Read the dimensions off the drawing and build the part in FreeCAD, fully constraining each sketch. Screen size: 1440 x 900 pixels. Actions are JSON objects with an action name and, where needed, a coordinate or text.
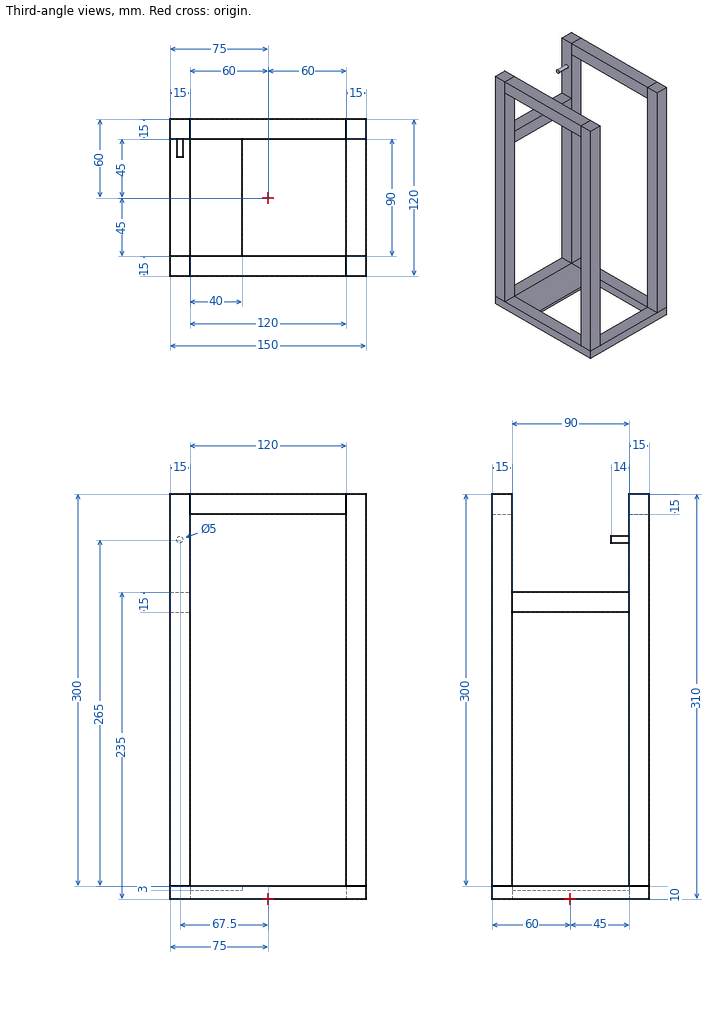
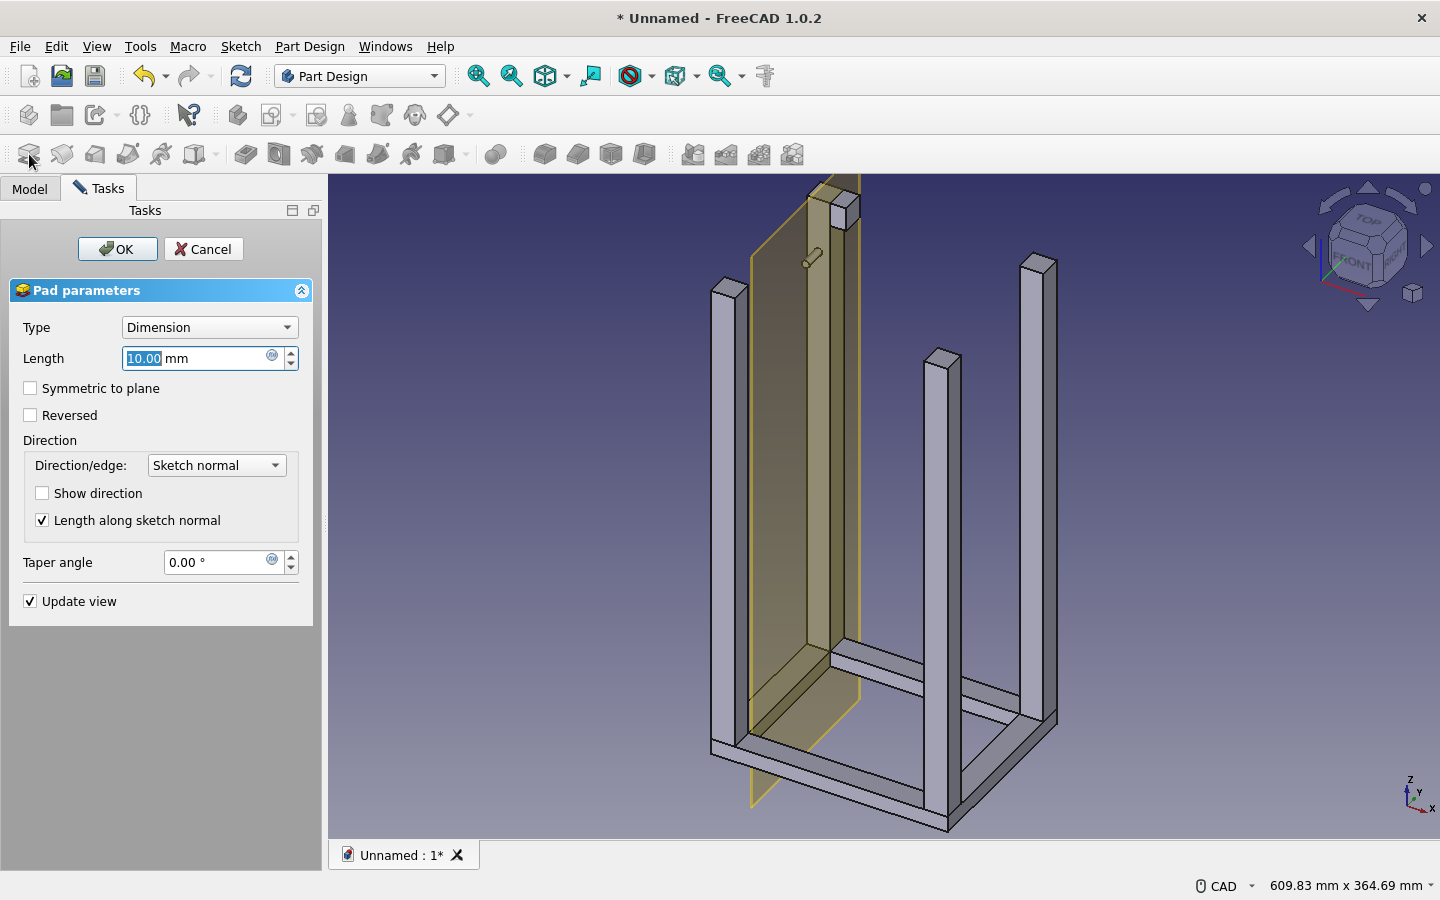
{"action": "type", "text": "120"}
{"action": "key", "text": "Tab"}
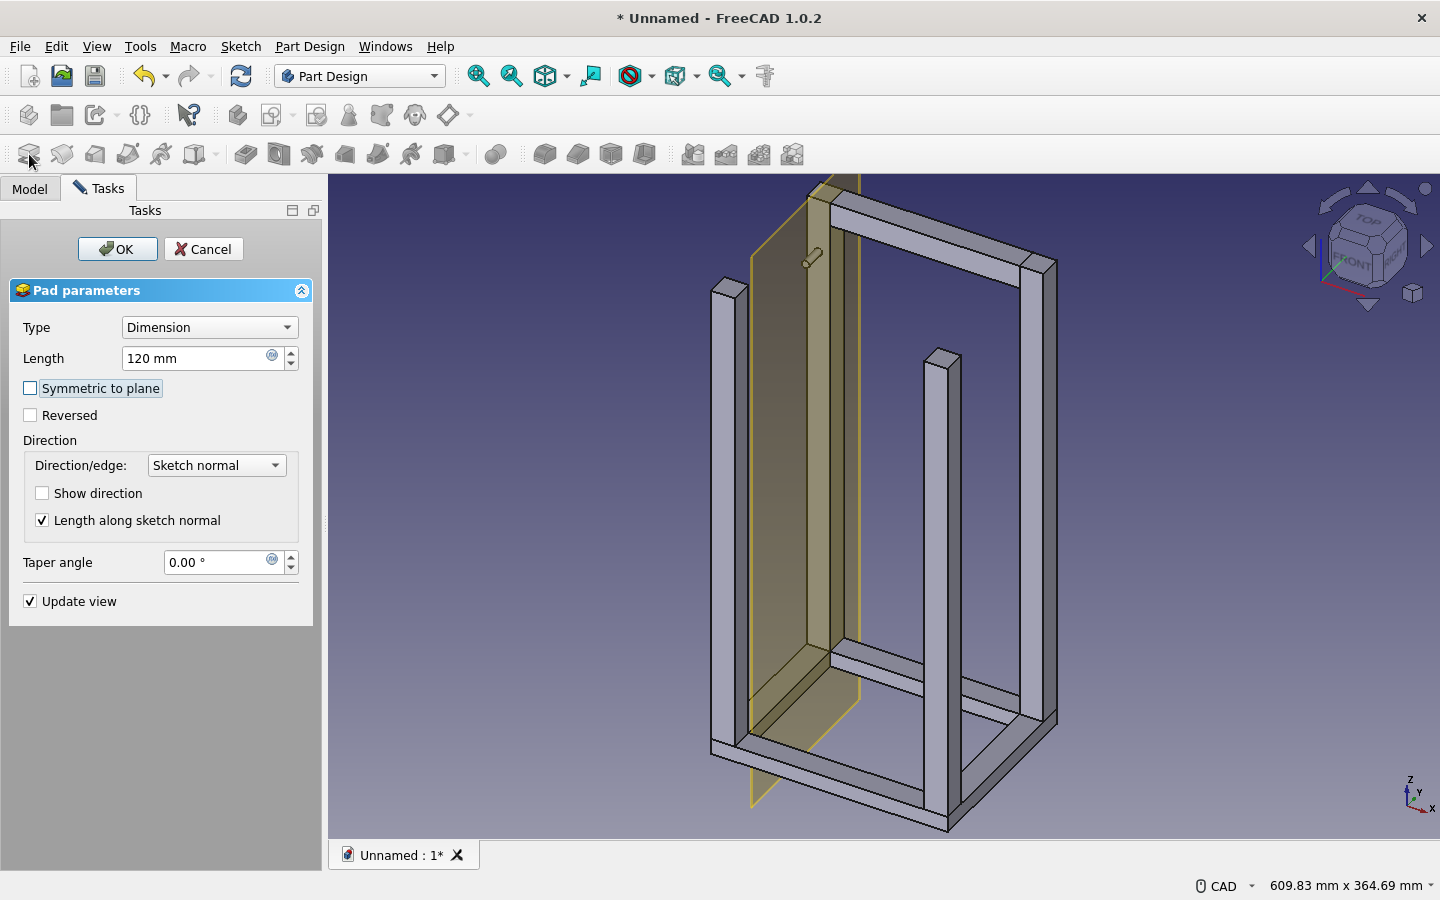
{"action": "left_click", "coordinate": [118, 249]}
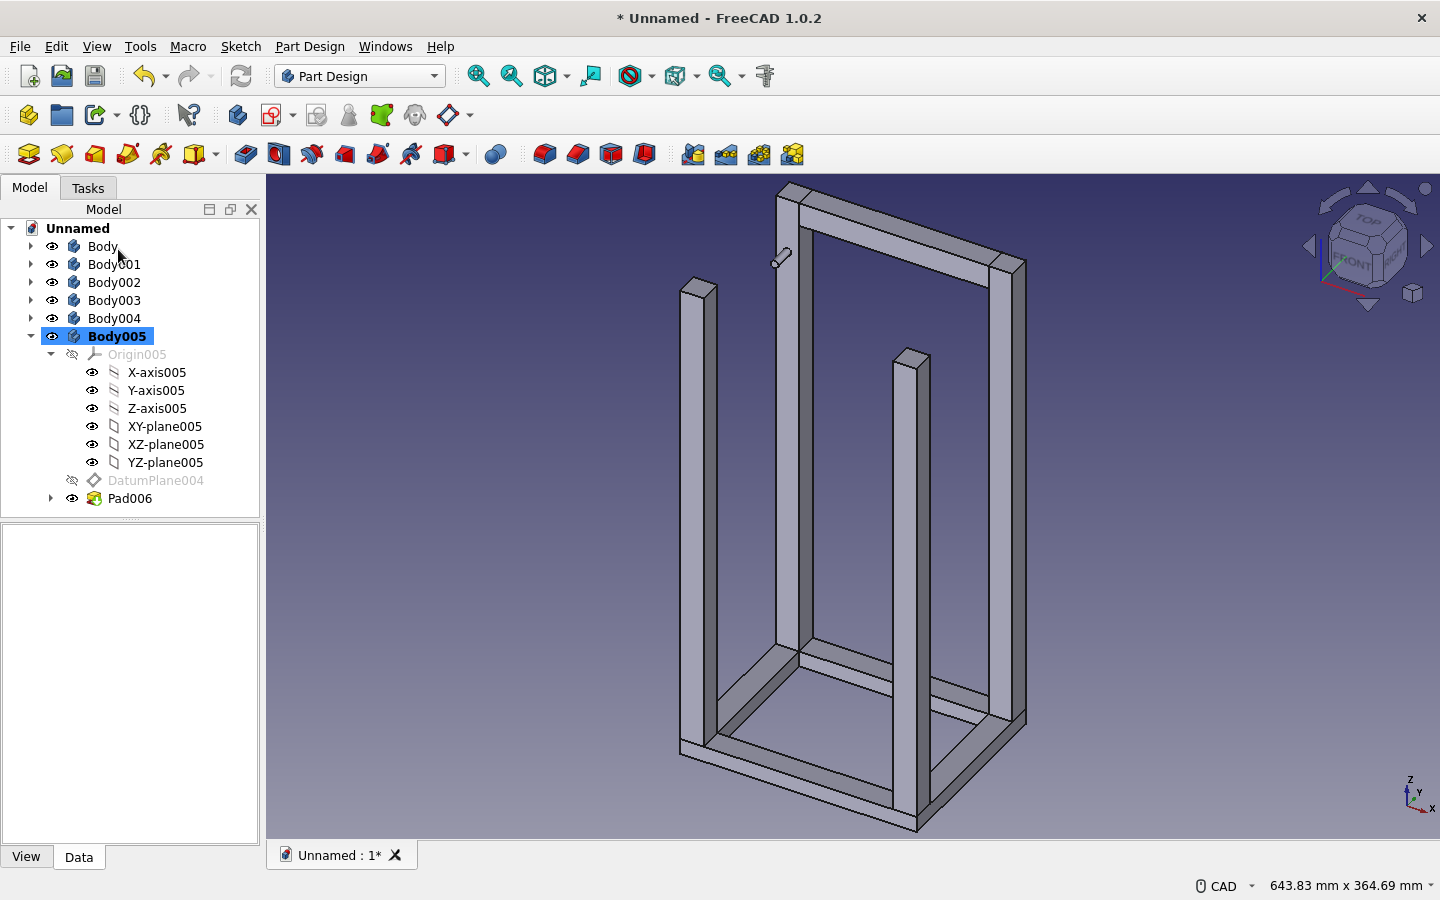
{"action": "left_click", "coordinate": [479, 76]}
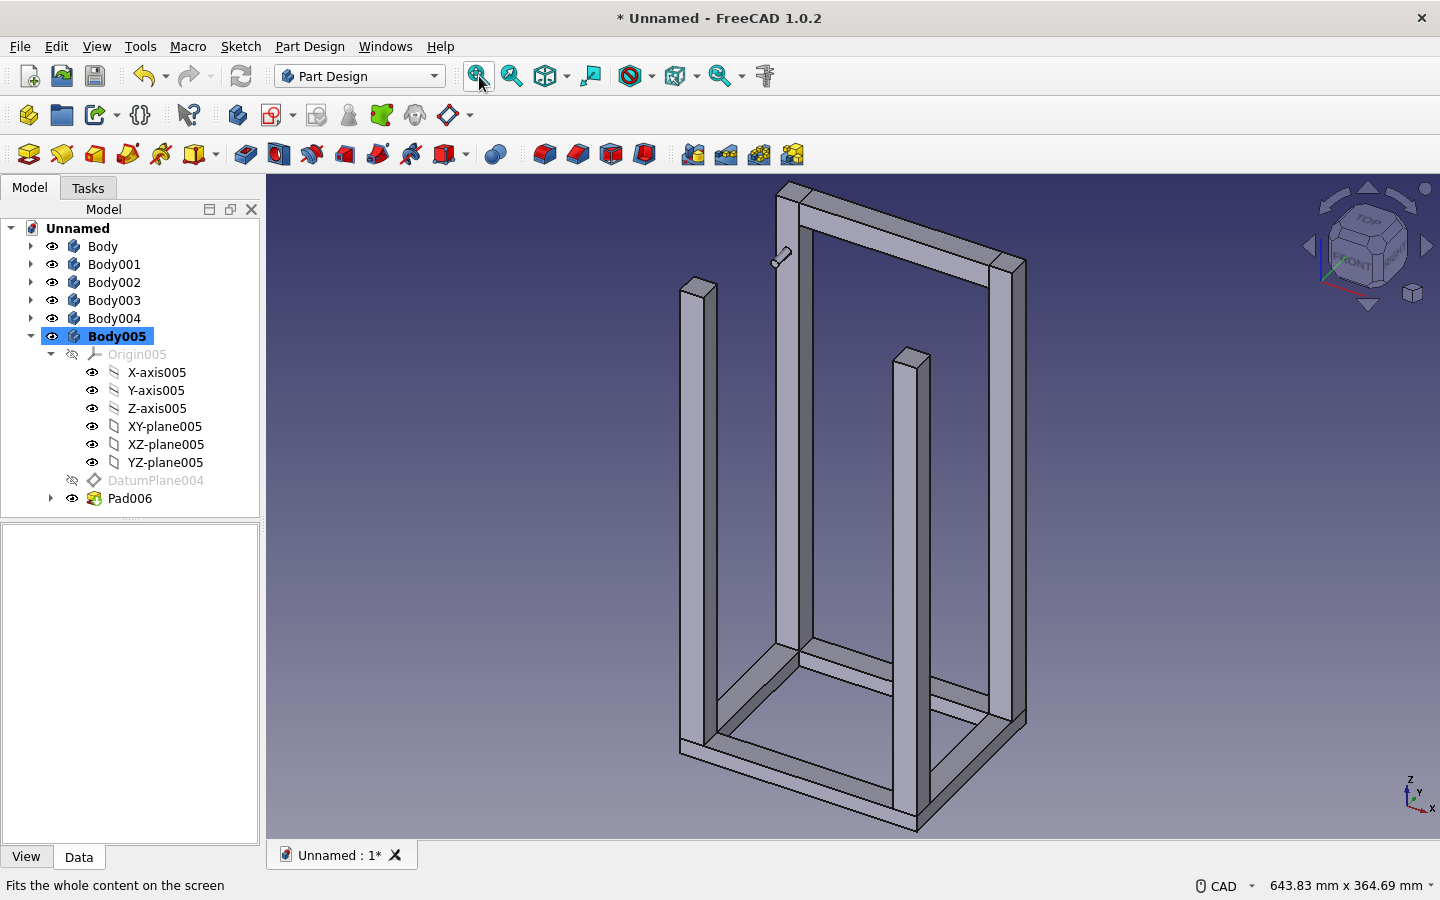
{"action": "left_click", "coordinate": [238, 116]}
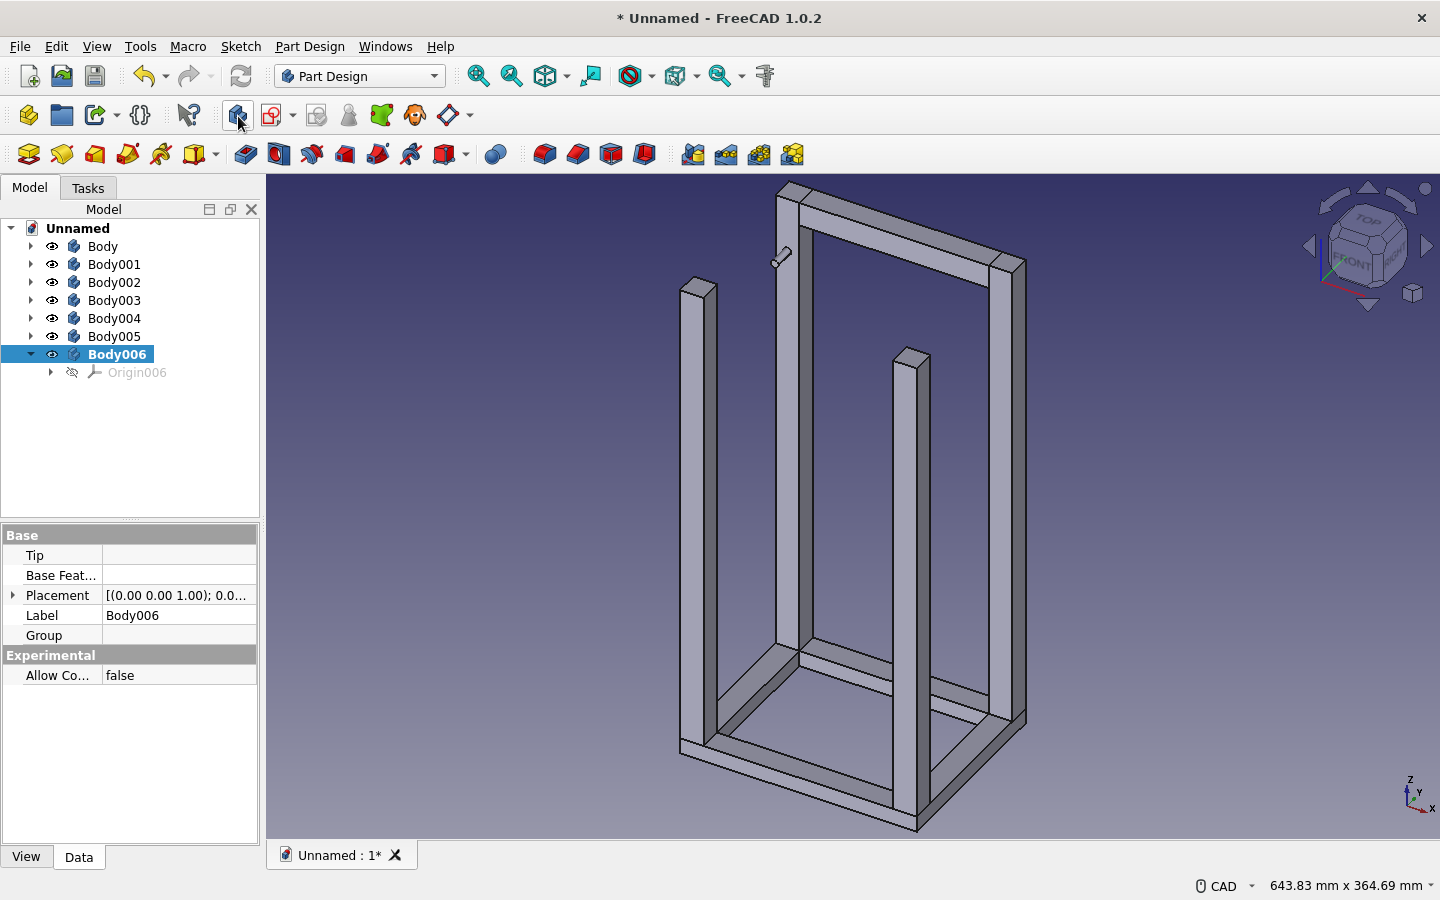
{"action": "left_click", "coordinate": [51, 372]}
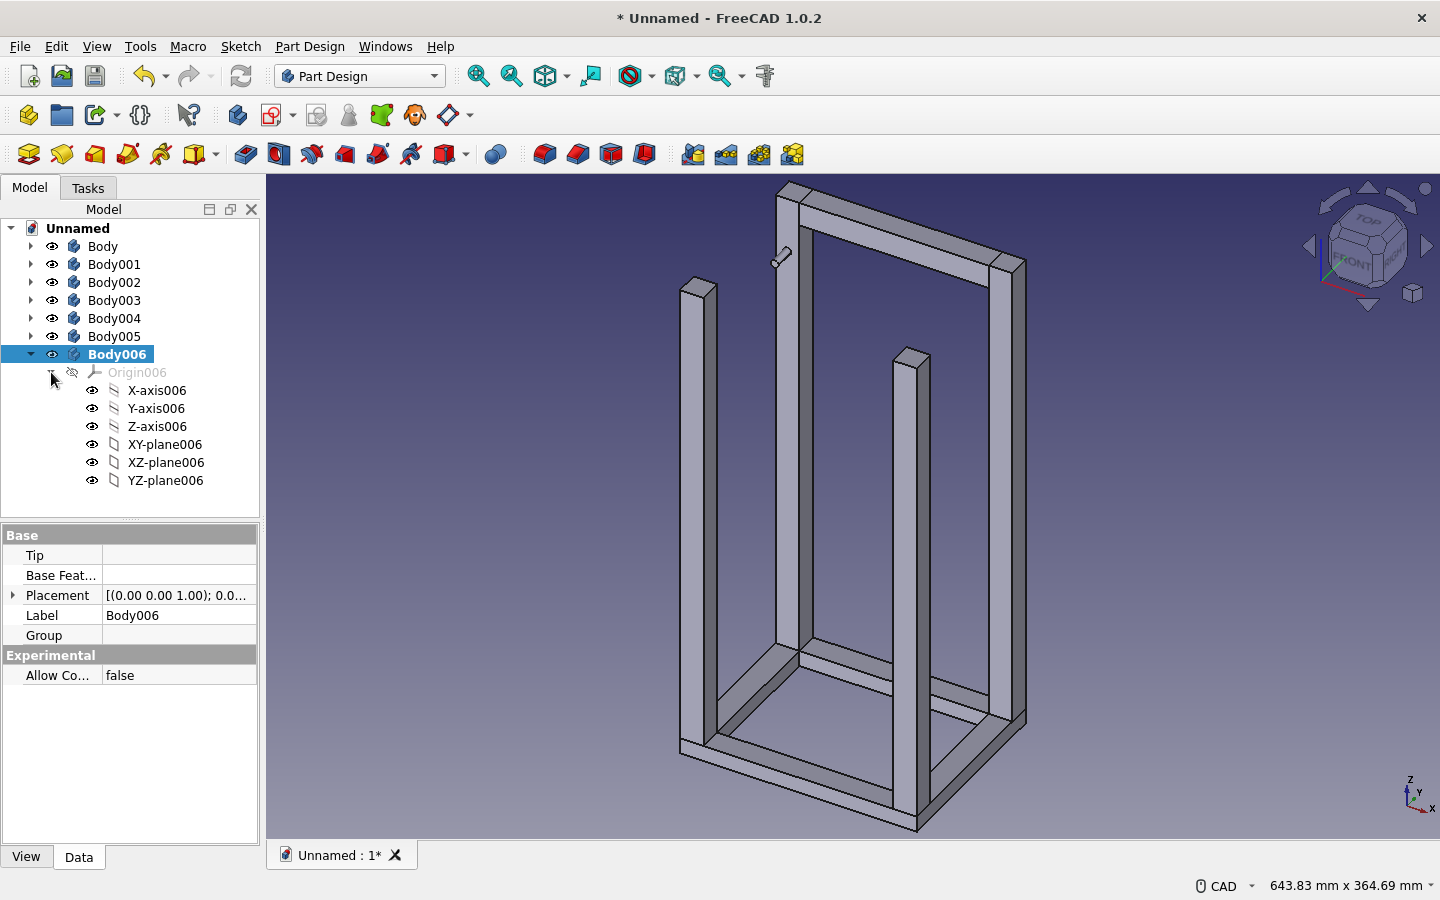
{"action": "left_click", "coordinate": [137, 480]}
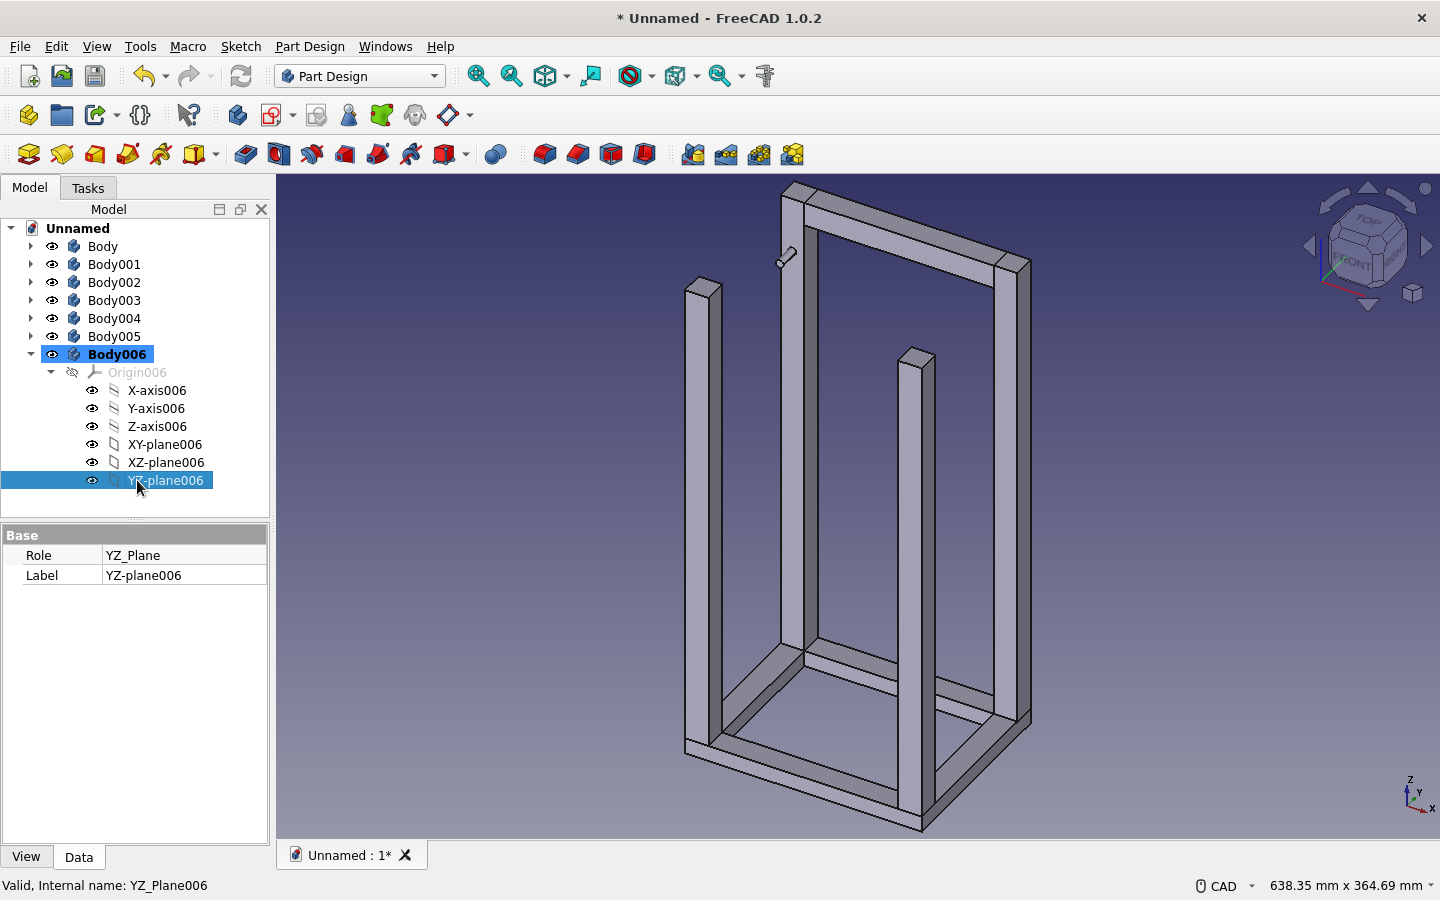
{"action": "left_click", "coordinate": [448, 116]}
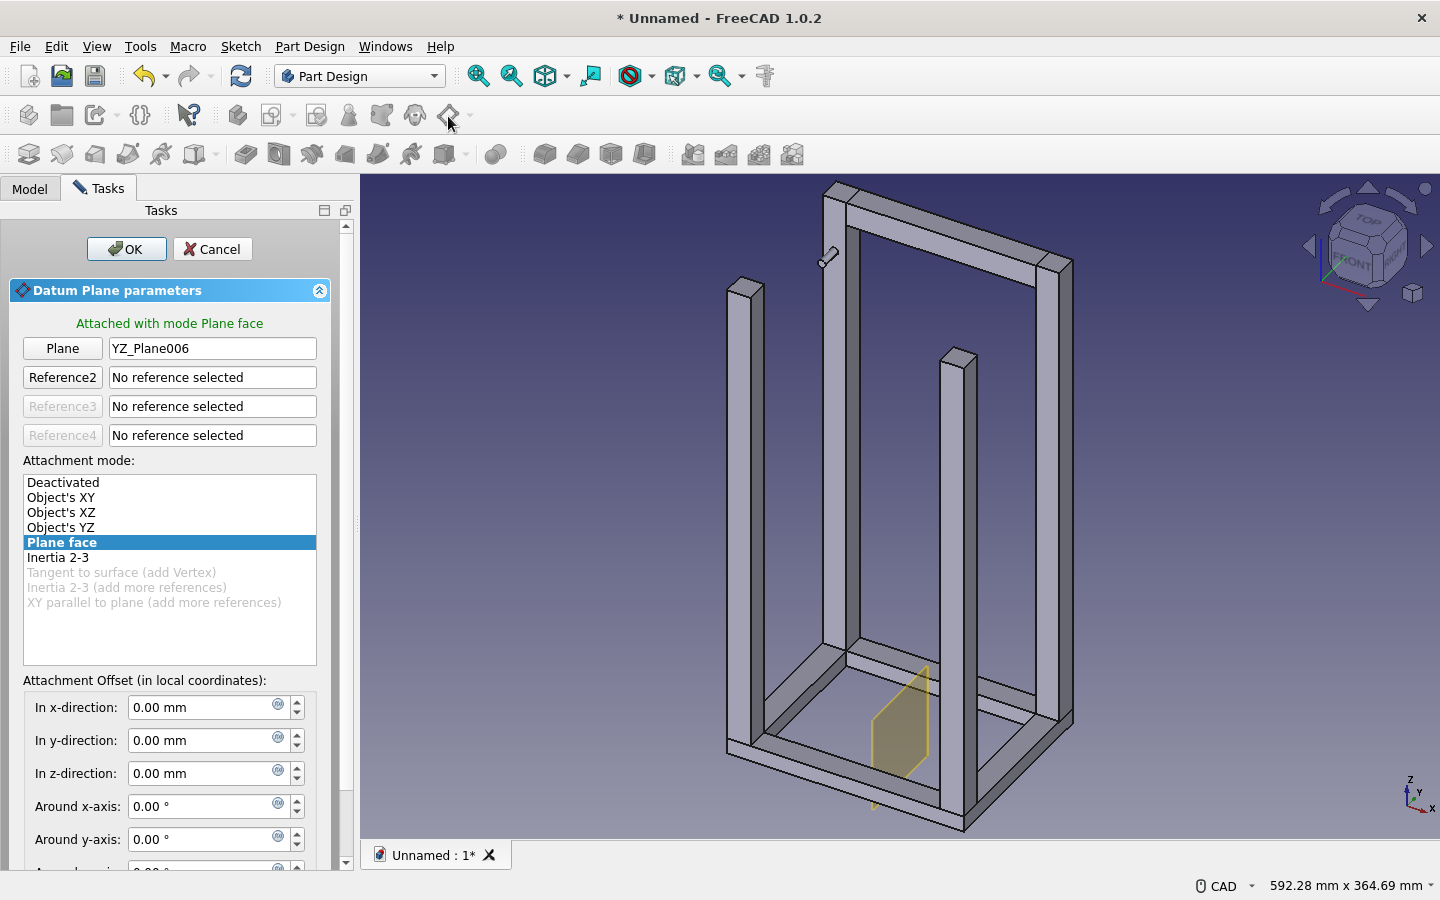
{"action": "triple_click", "coordinate": [210, 774]}